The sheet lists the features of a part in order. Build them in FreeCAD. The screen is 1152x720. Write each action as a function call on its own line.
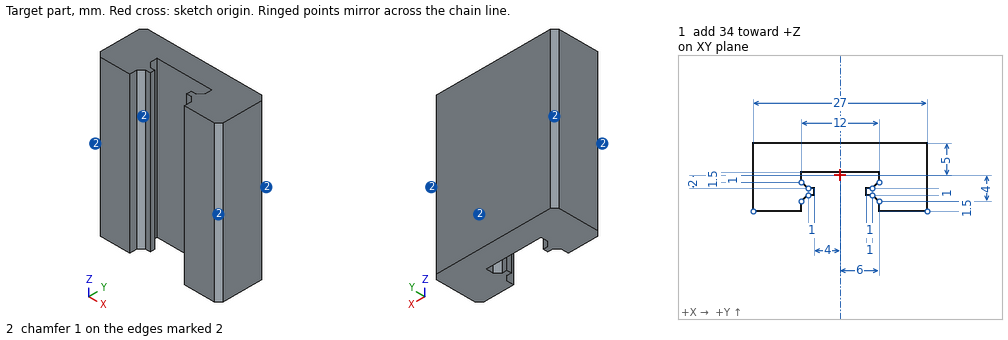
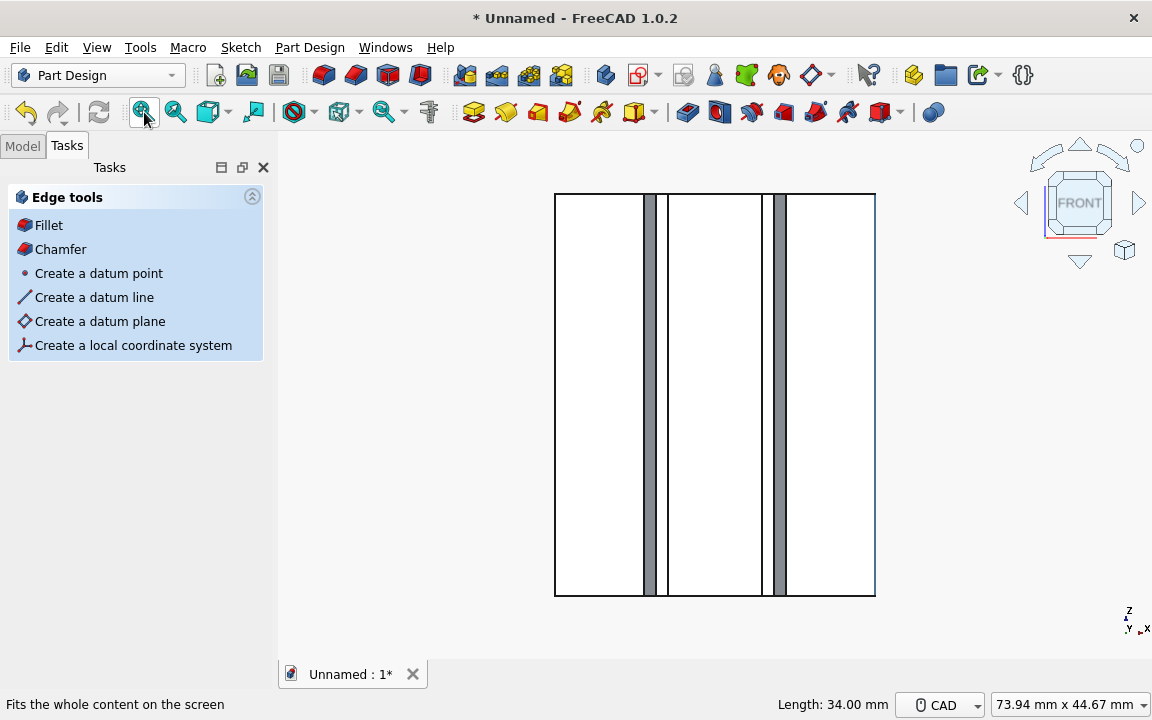
click(555, 394, ctrl)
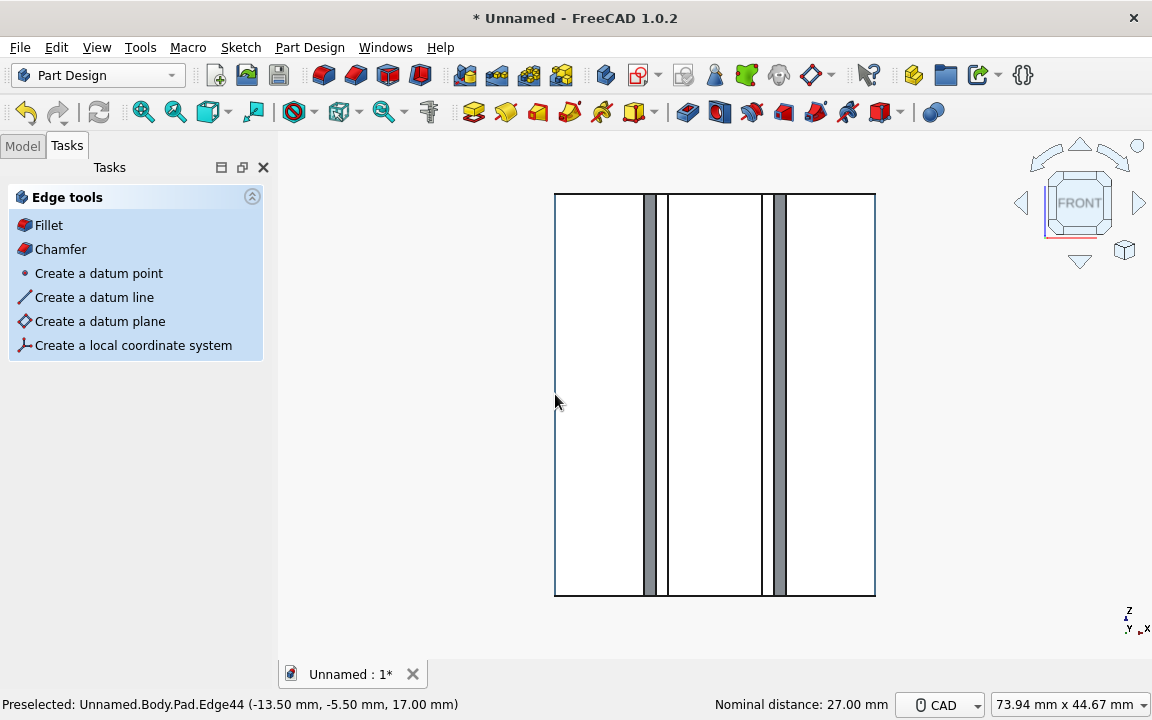
key(3)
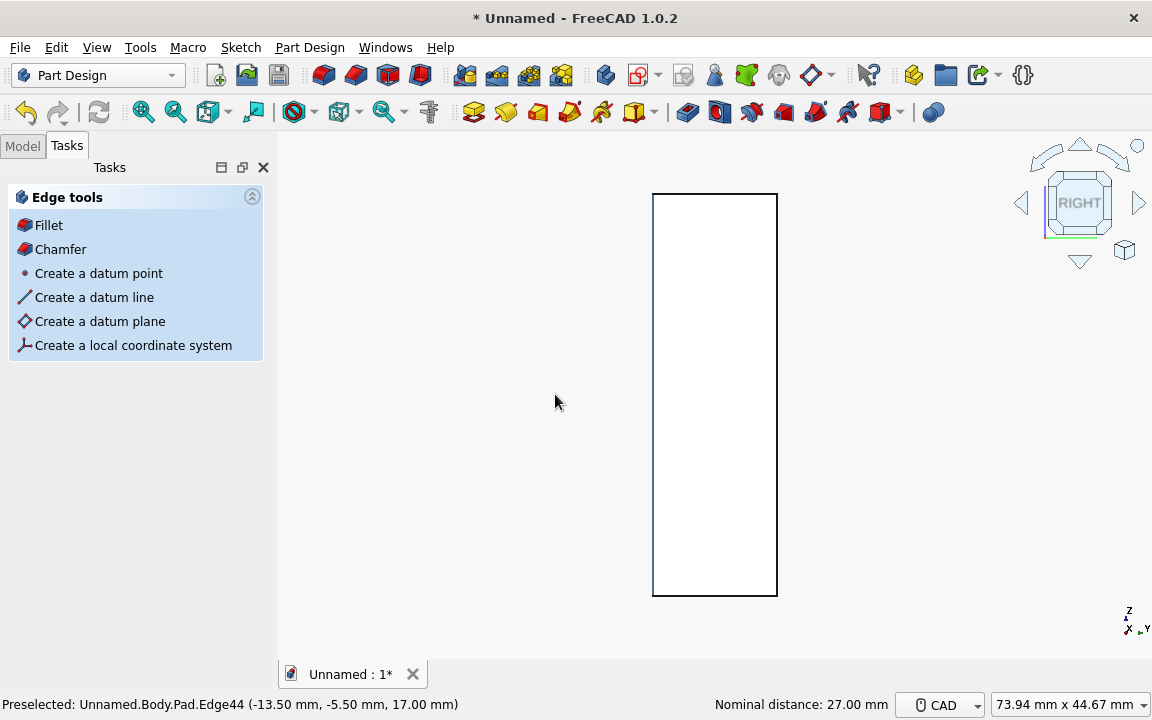
click(777, 394, ctrl)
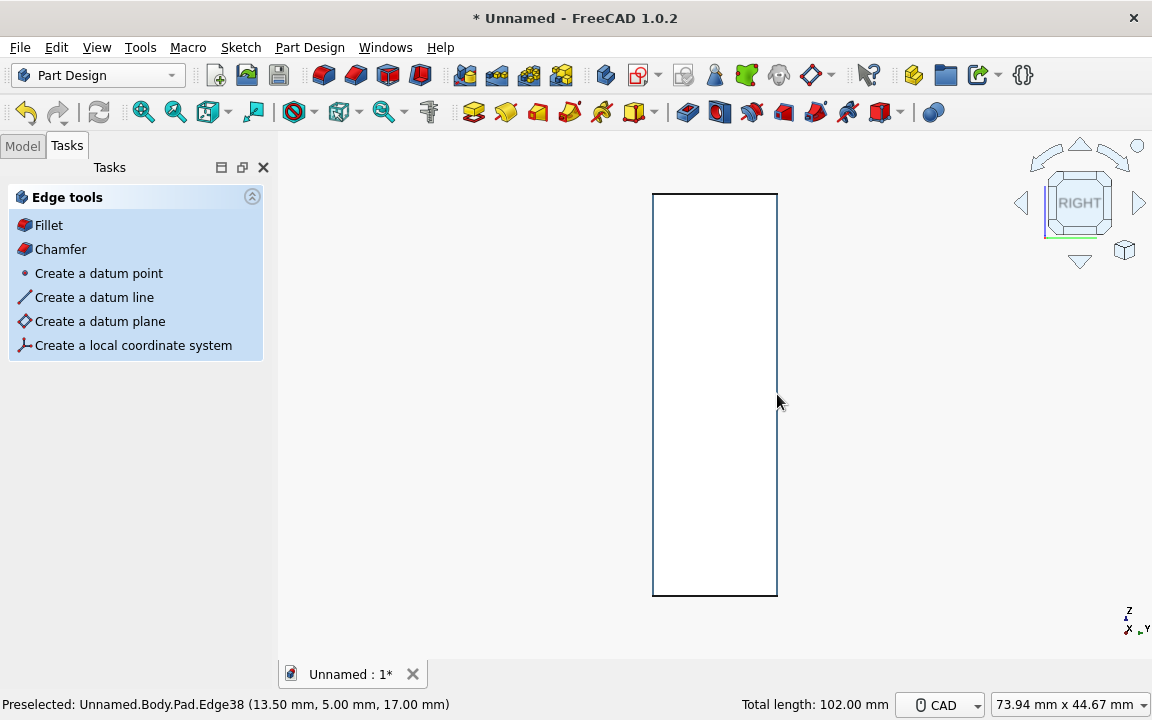
key(5)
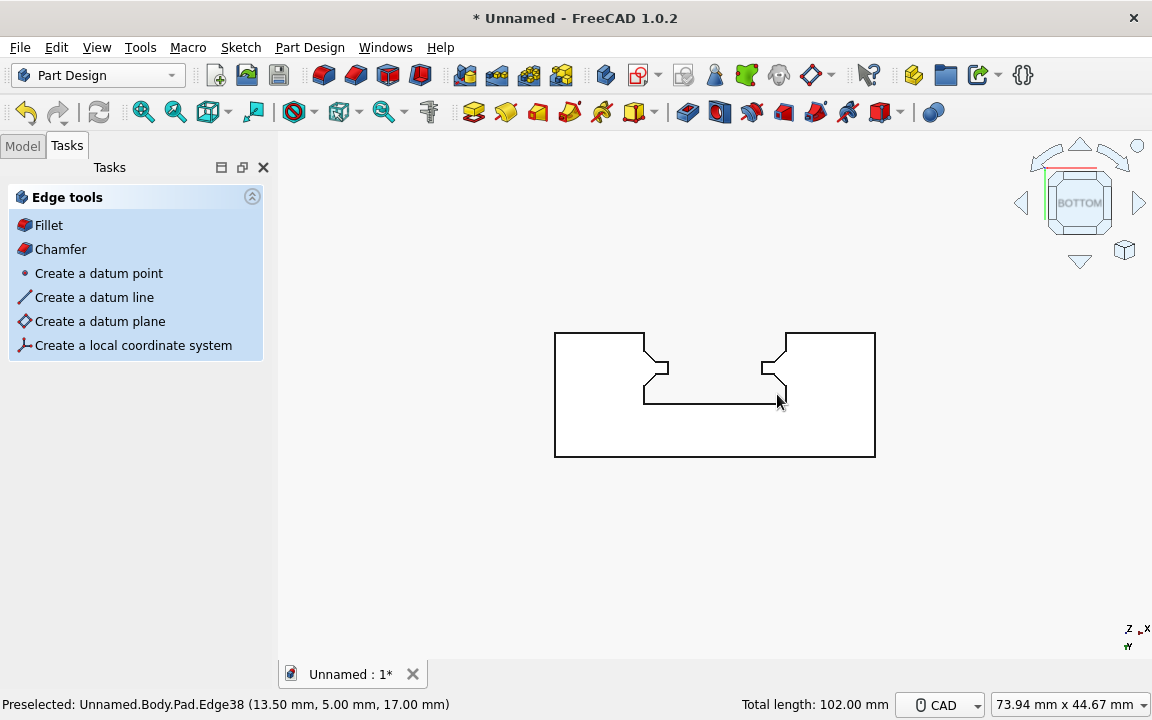
key(v)
key(f)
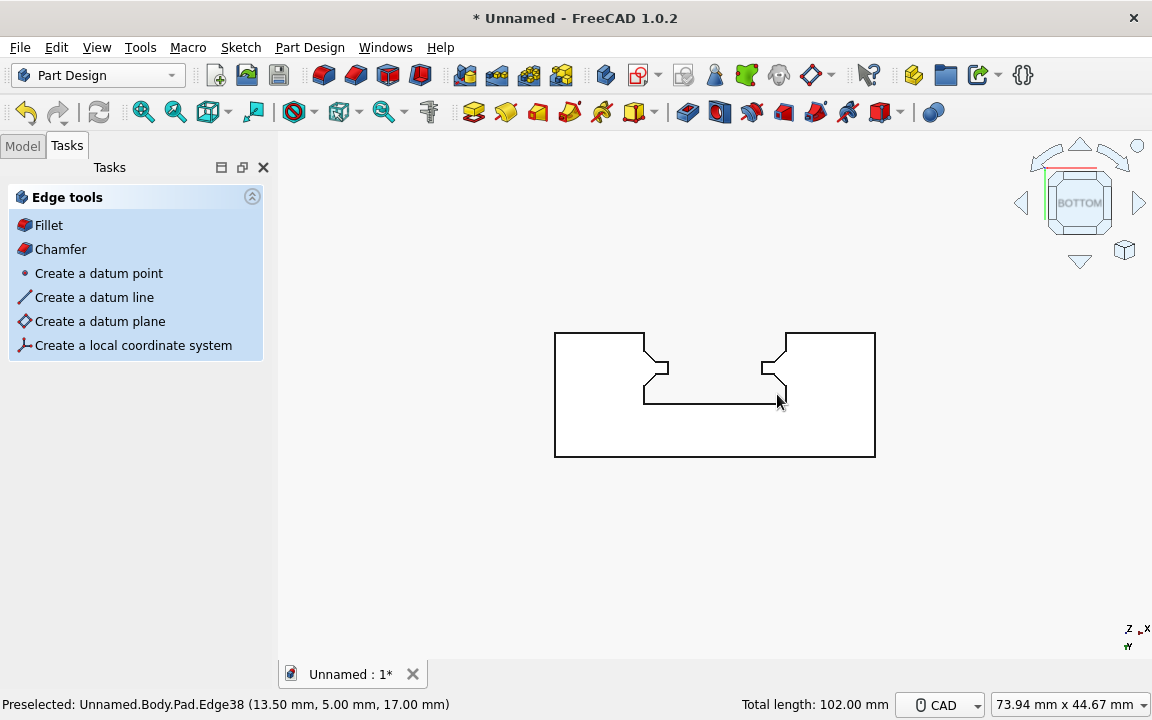
key(4)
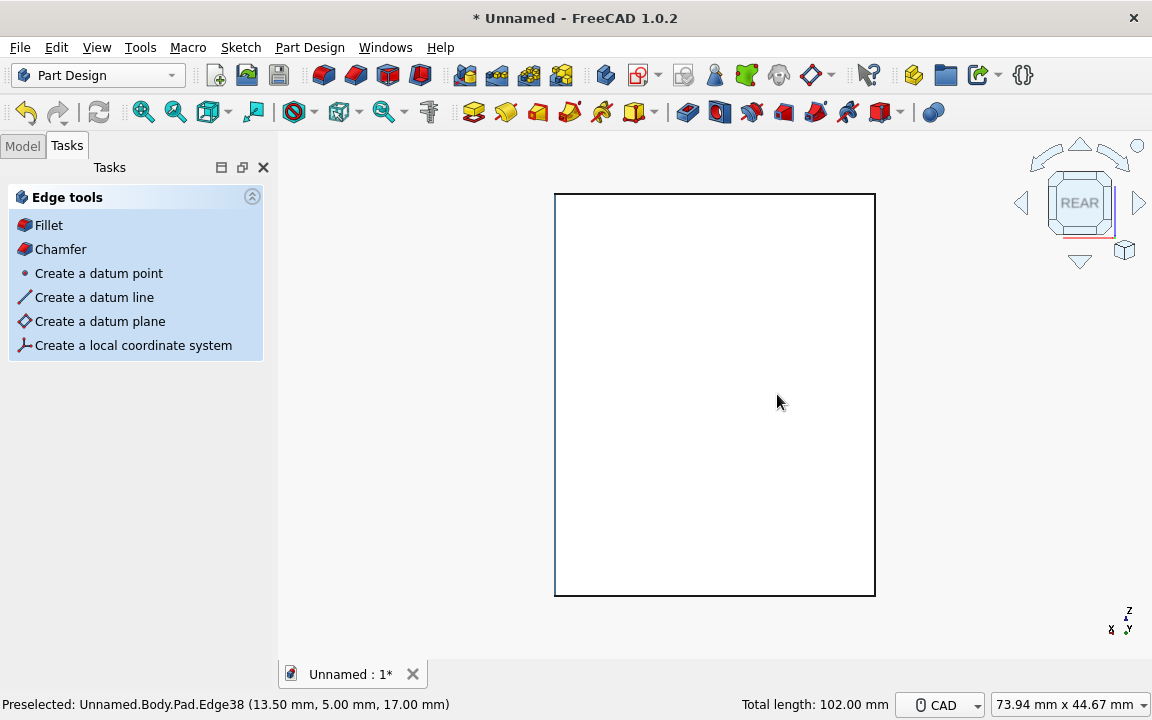
click(875, 394, ctrl)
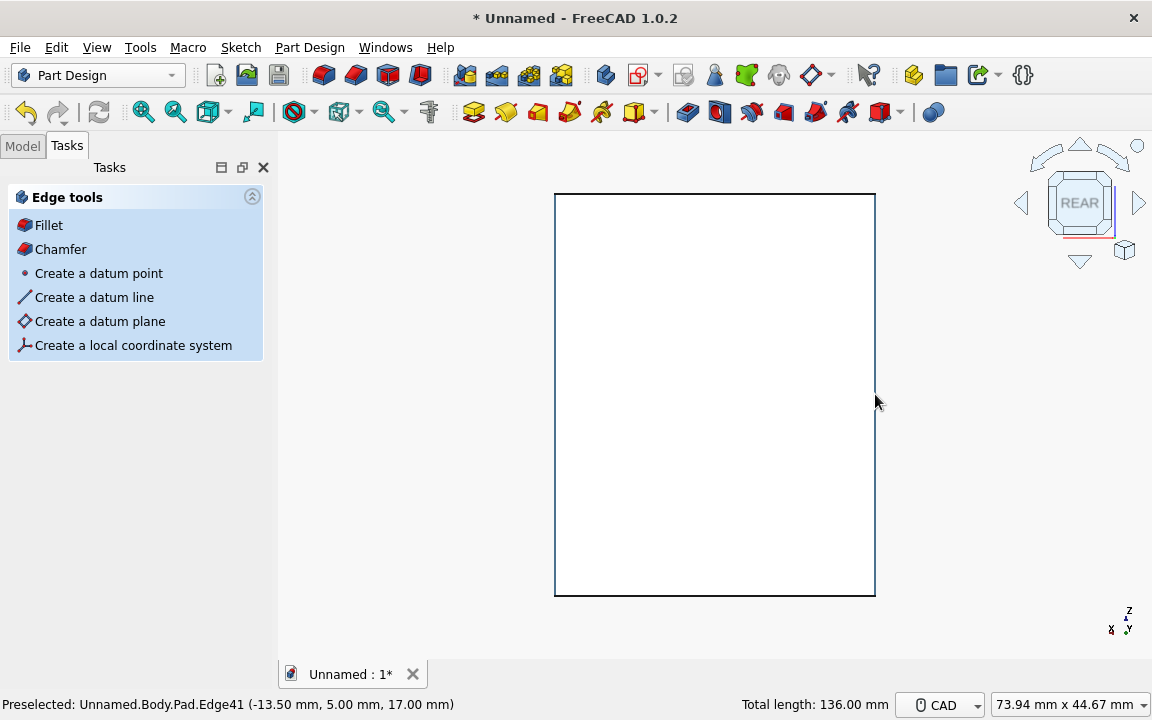
click(356, 76)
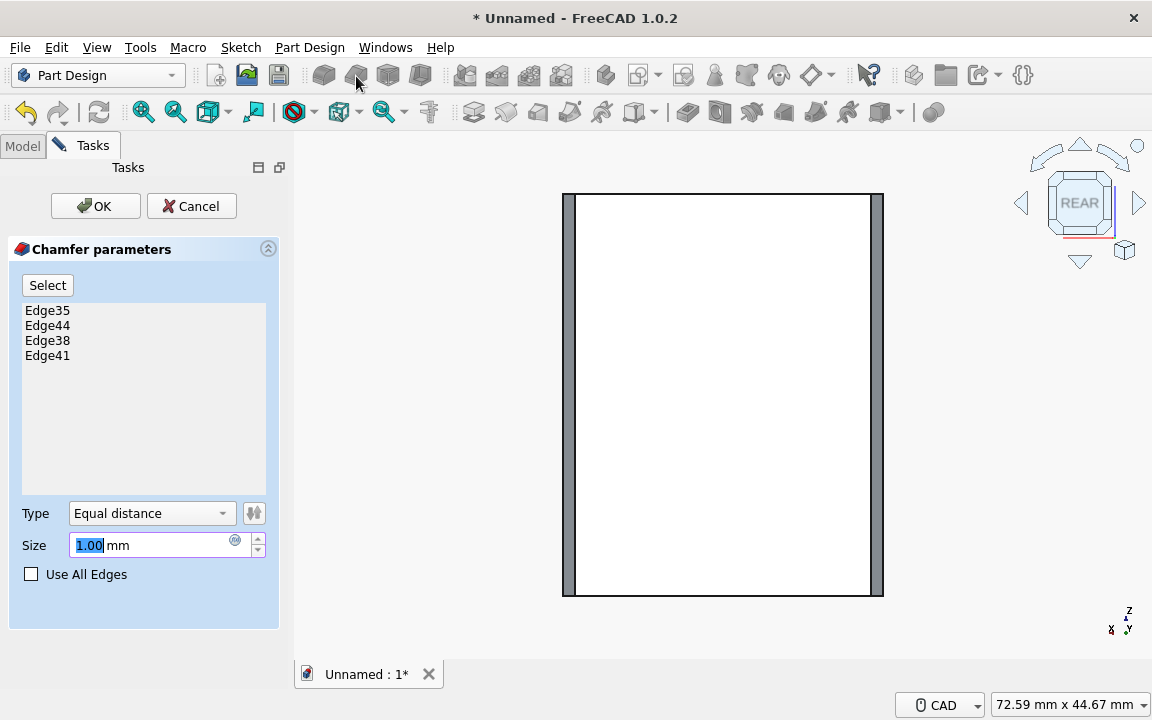
text(1)
key(Tab)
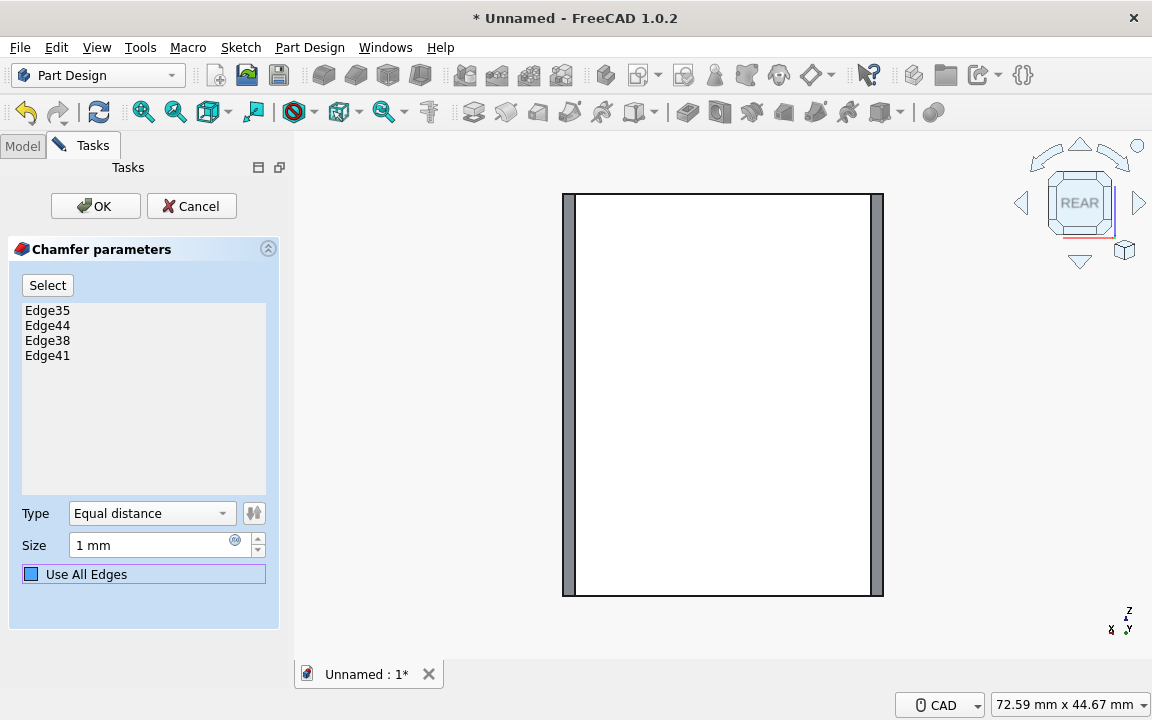
click(96, 206)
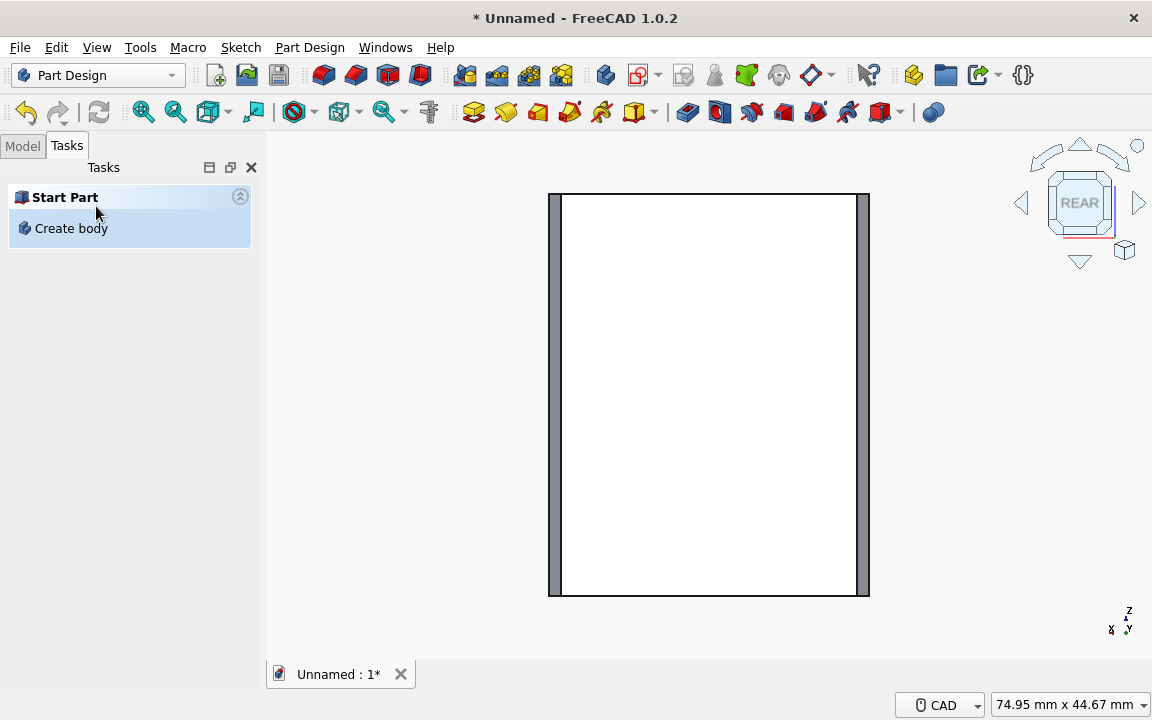
key(0)